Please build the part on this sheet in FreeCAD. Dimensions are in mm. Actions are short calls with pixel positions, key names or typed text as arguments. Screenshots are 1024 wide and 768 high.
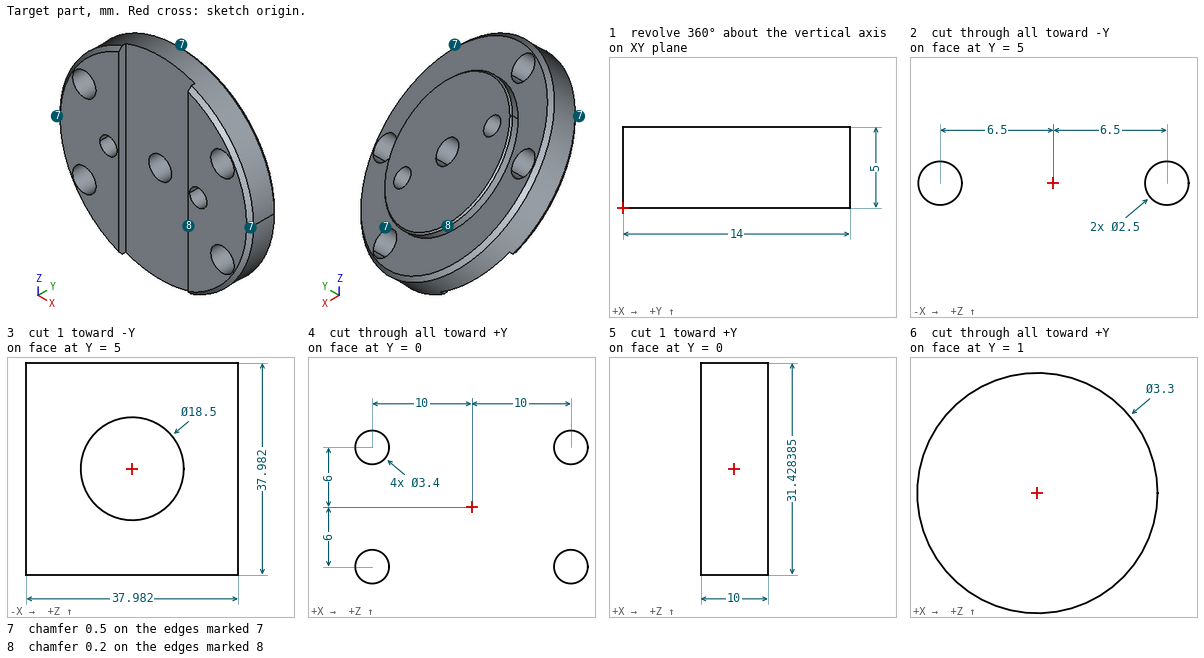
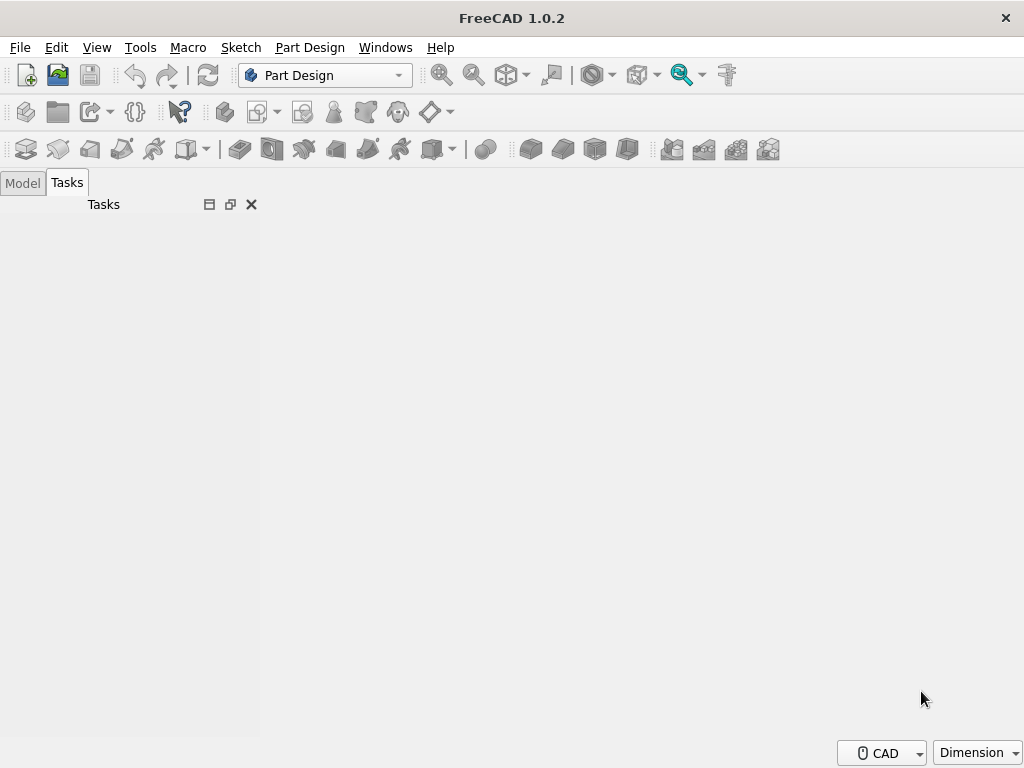
key(ctrl+n)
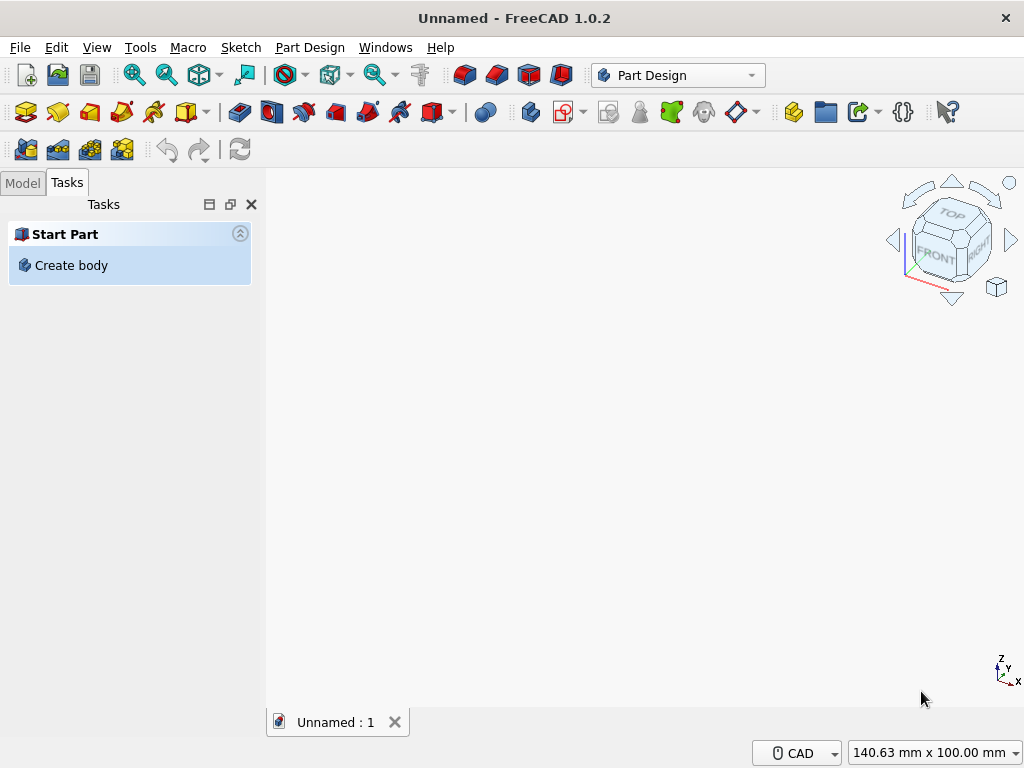
click(564, 112)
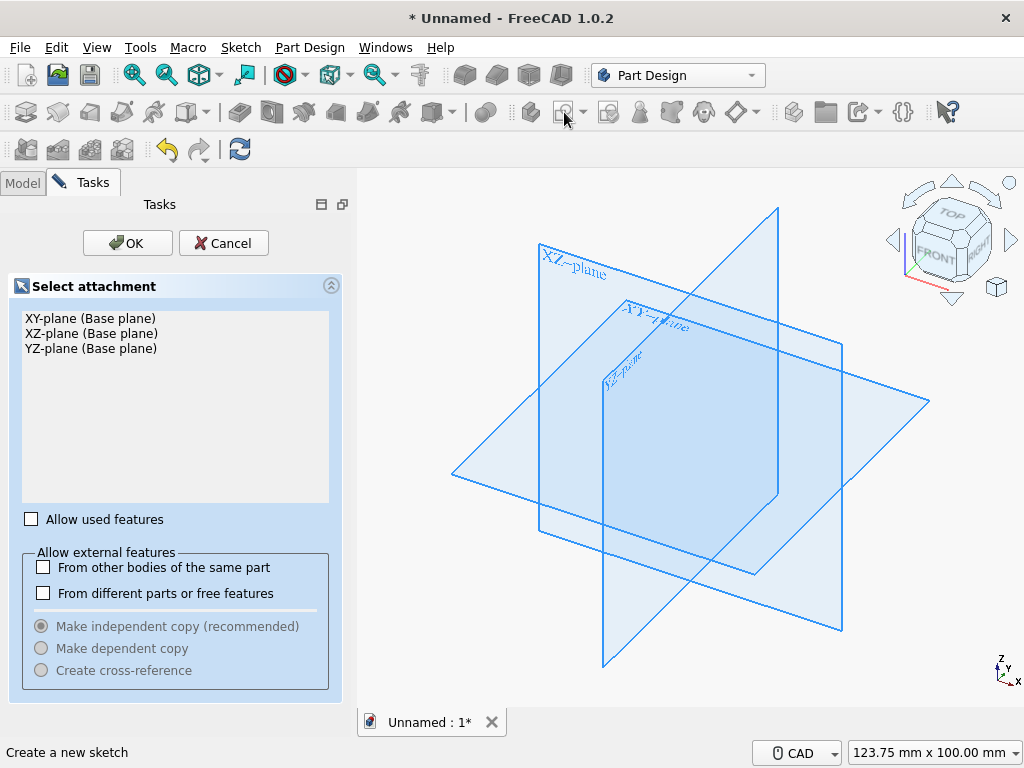
click(82, 318)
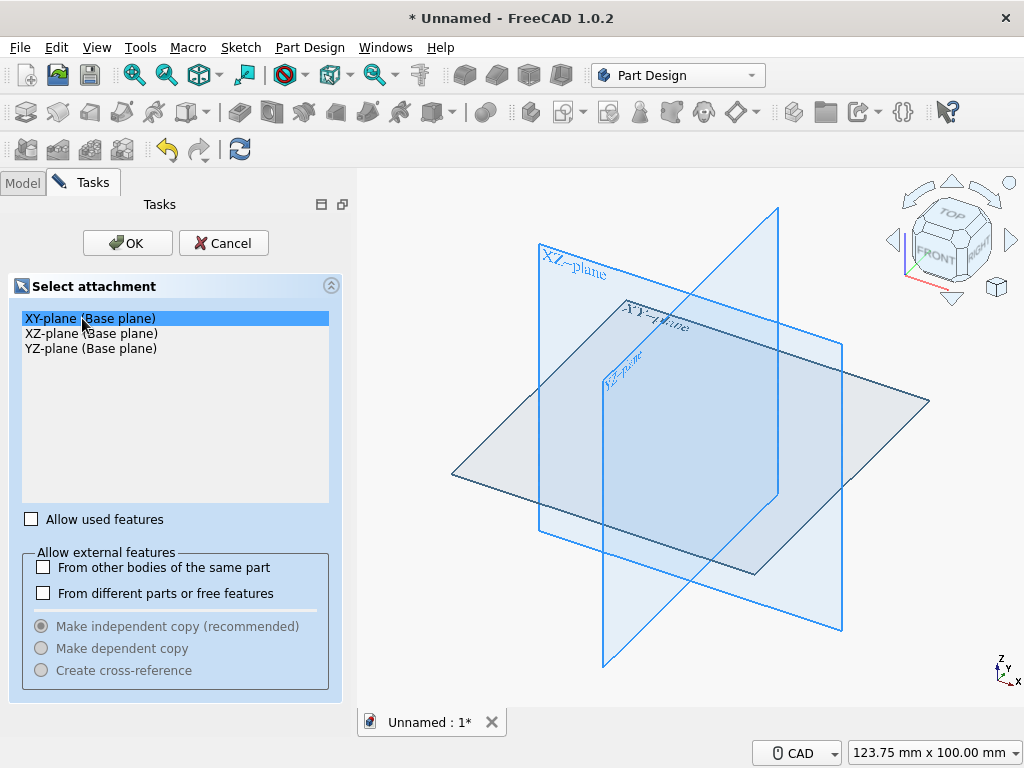
click(128, 243)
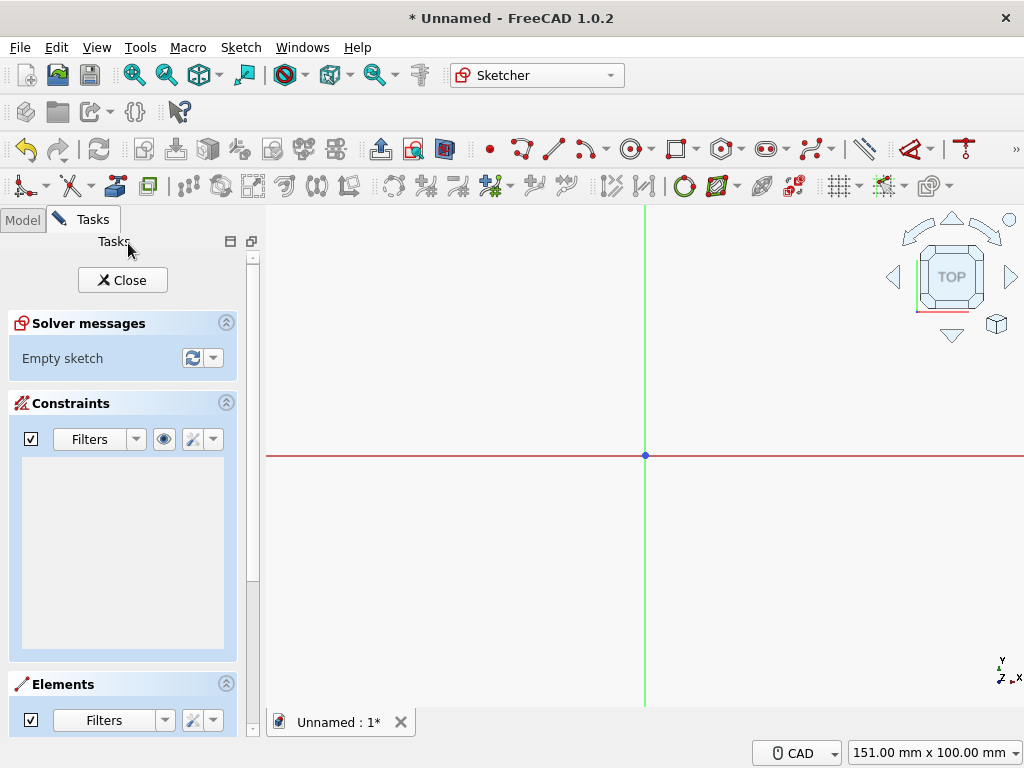
scroll(701, 441, up, 9)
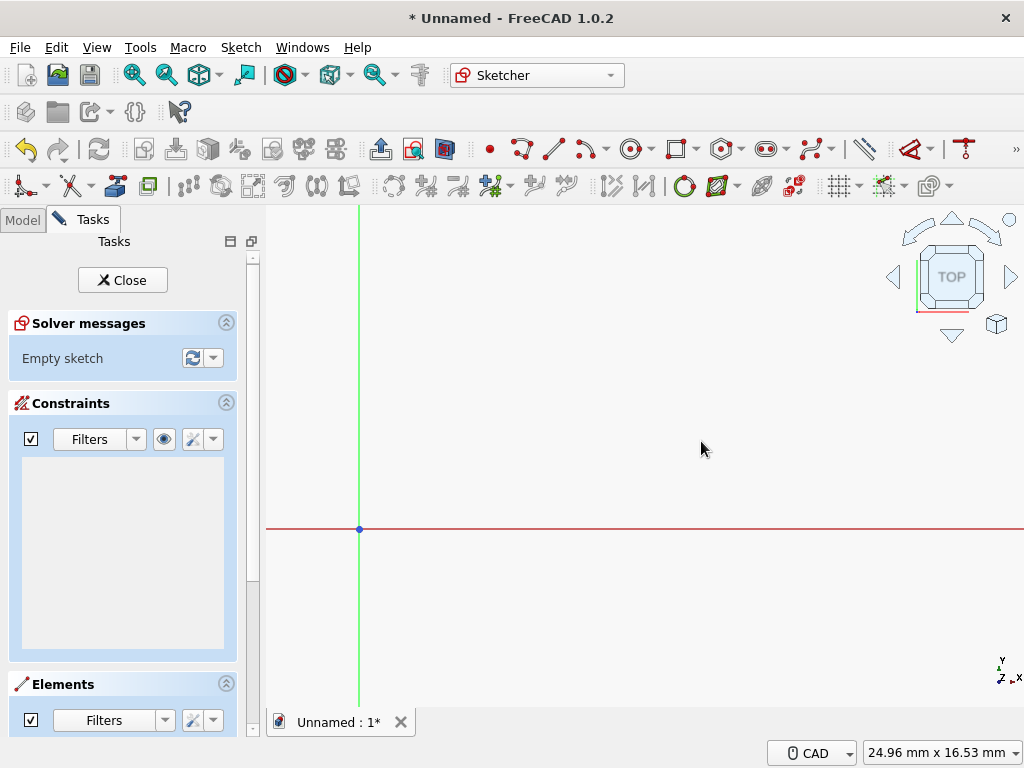
key(g)
key(r)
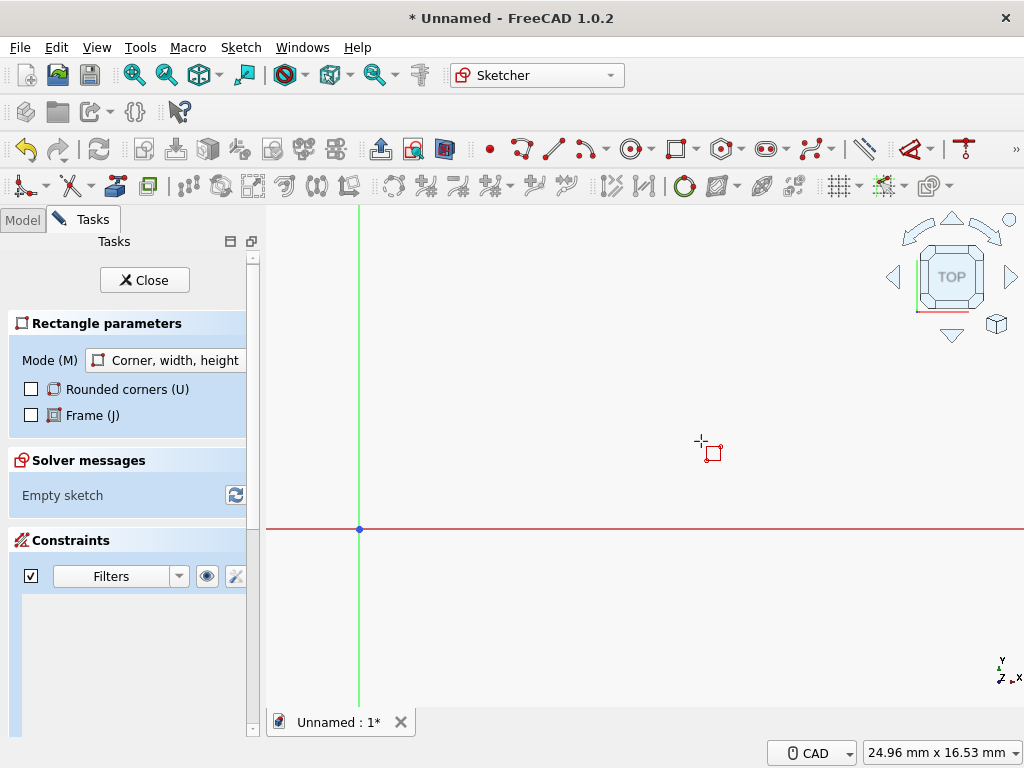
click(359, 529)
click(784, 378)
key(Escape)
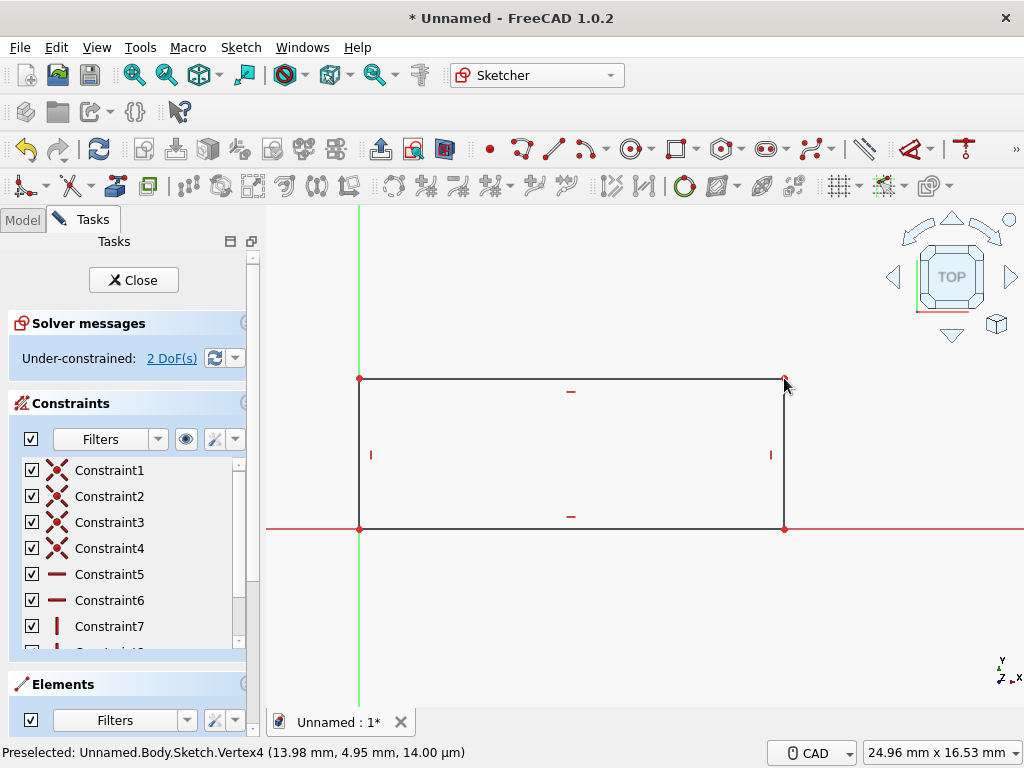
click(910, 150)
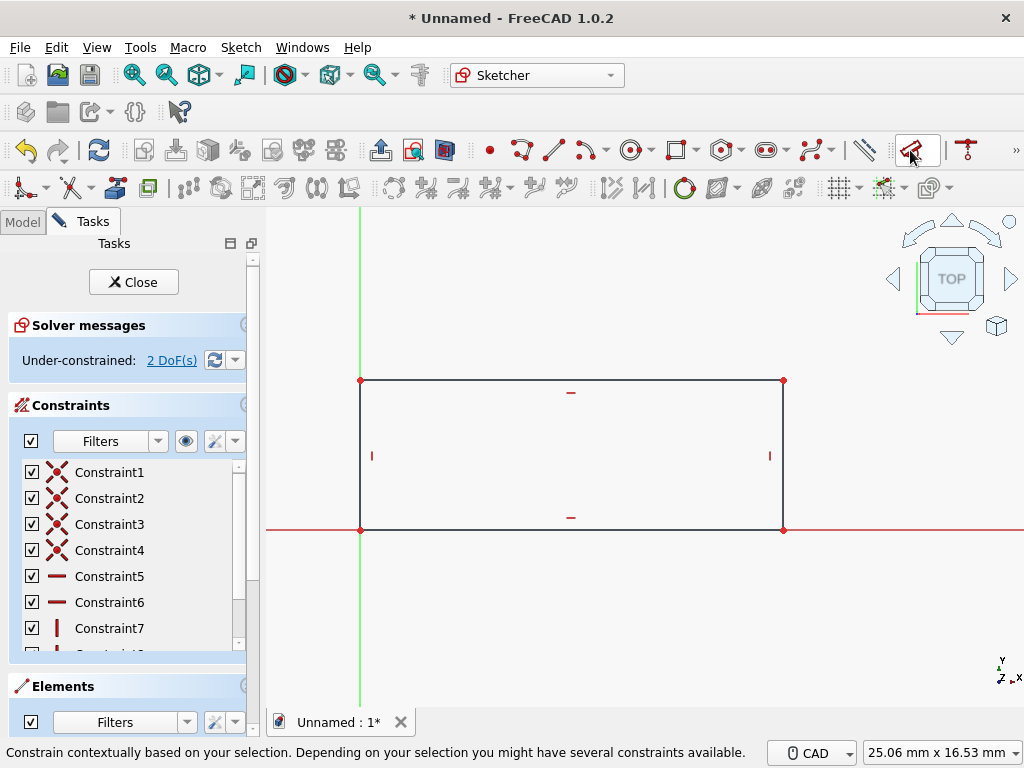
click(783, 485)
click(817, 455)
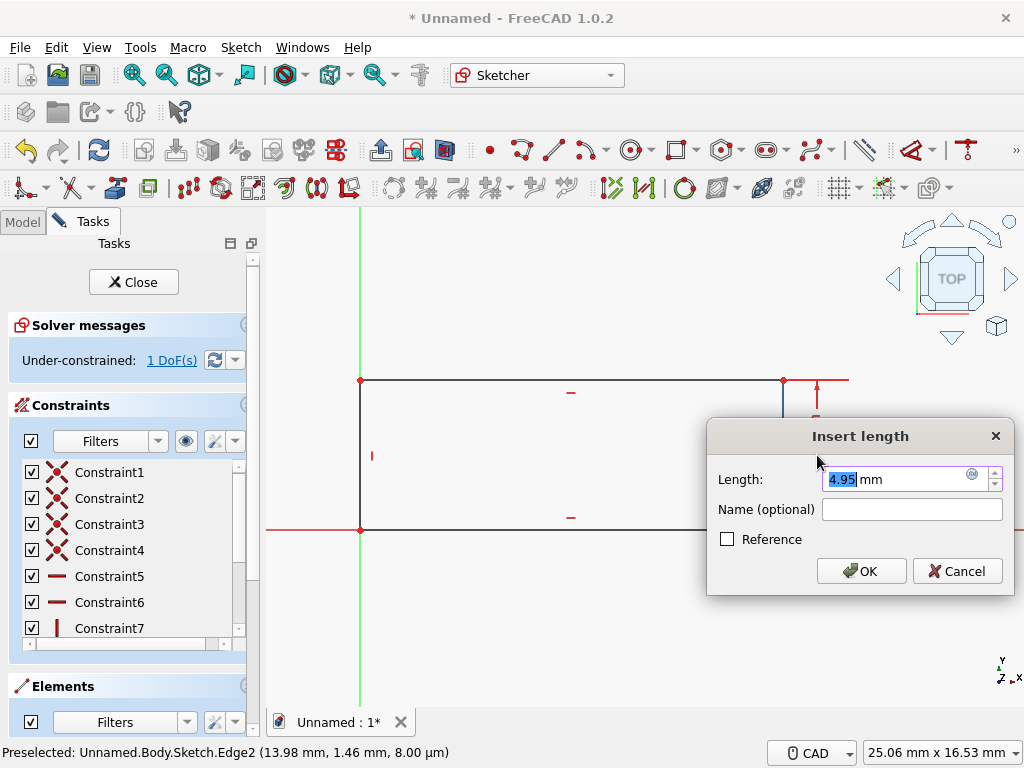
text(5)
key(Return)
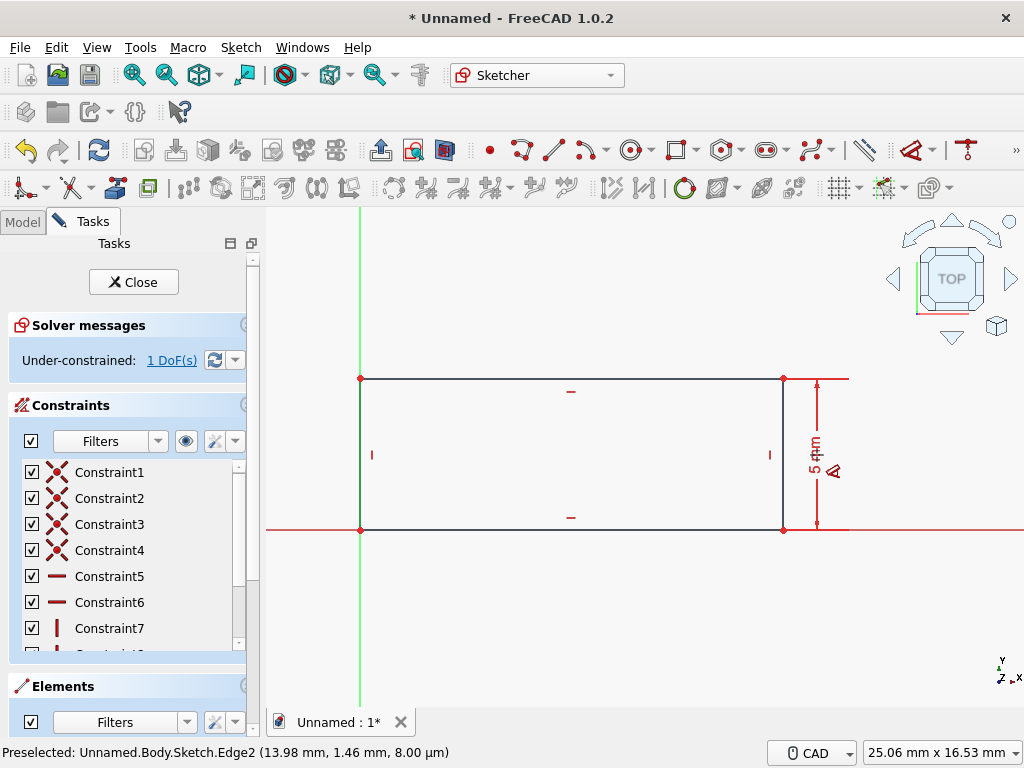
click(487, 530)
click(572, 564)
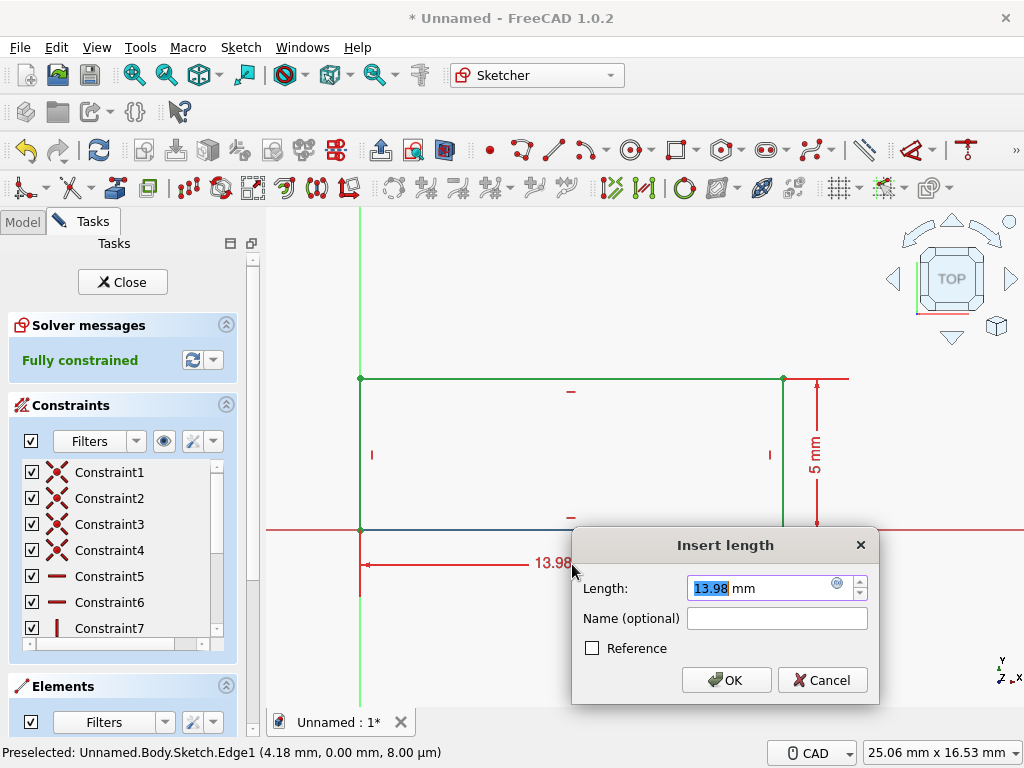
text(14)
key(Return)
key(Escape)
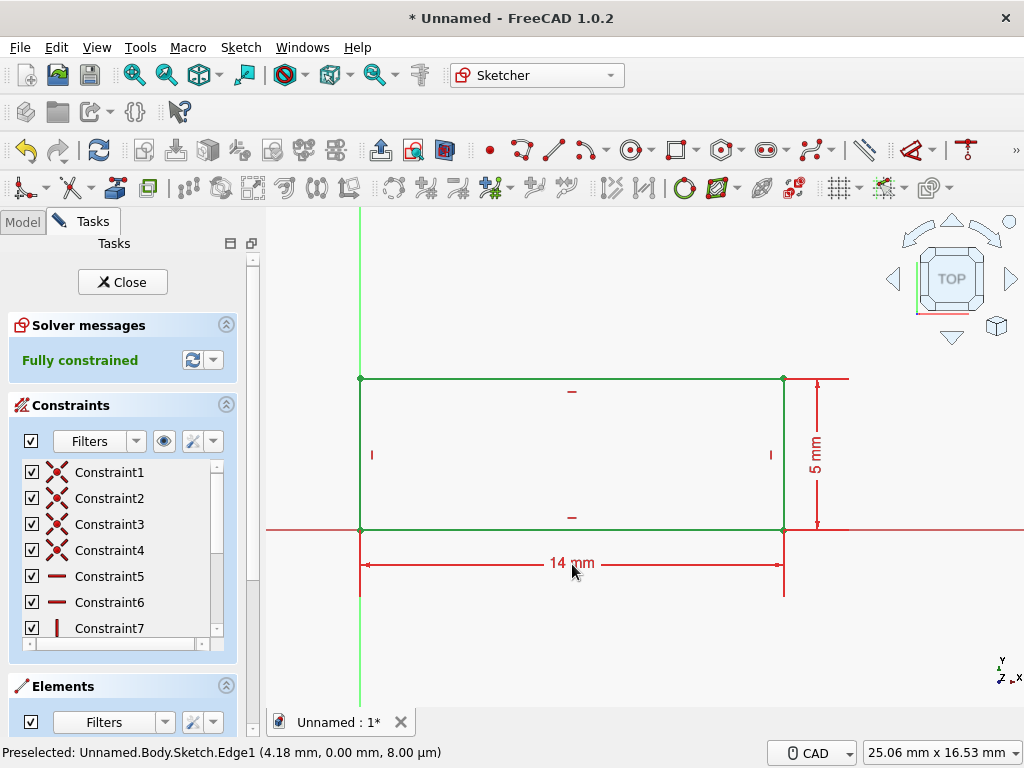
click(123, 282)